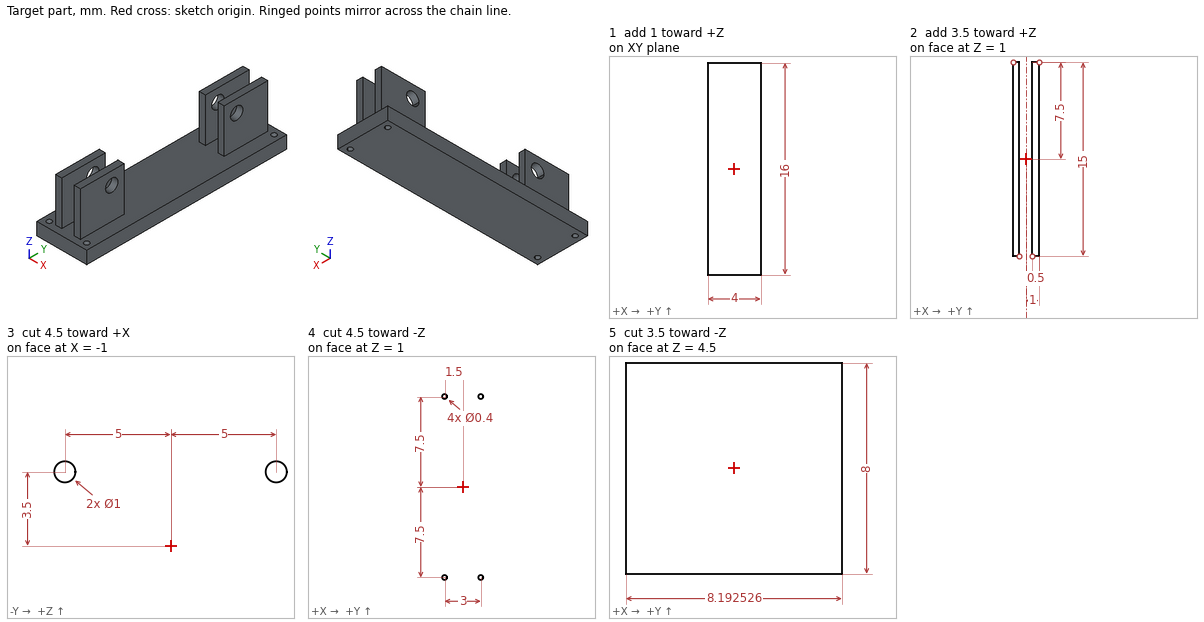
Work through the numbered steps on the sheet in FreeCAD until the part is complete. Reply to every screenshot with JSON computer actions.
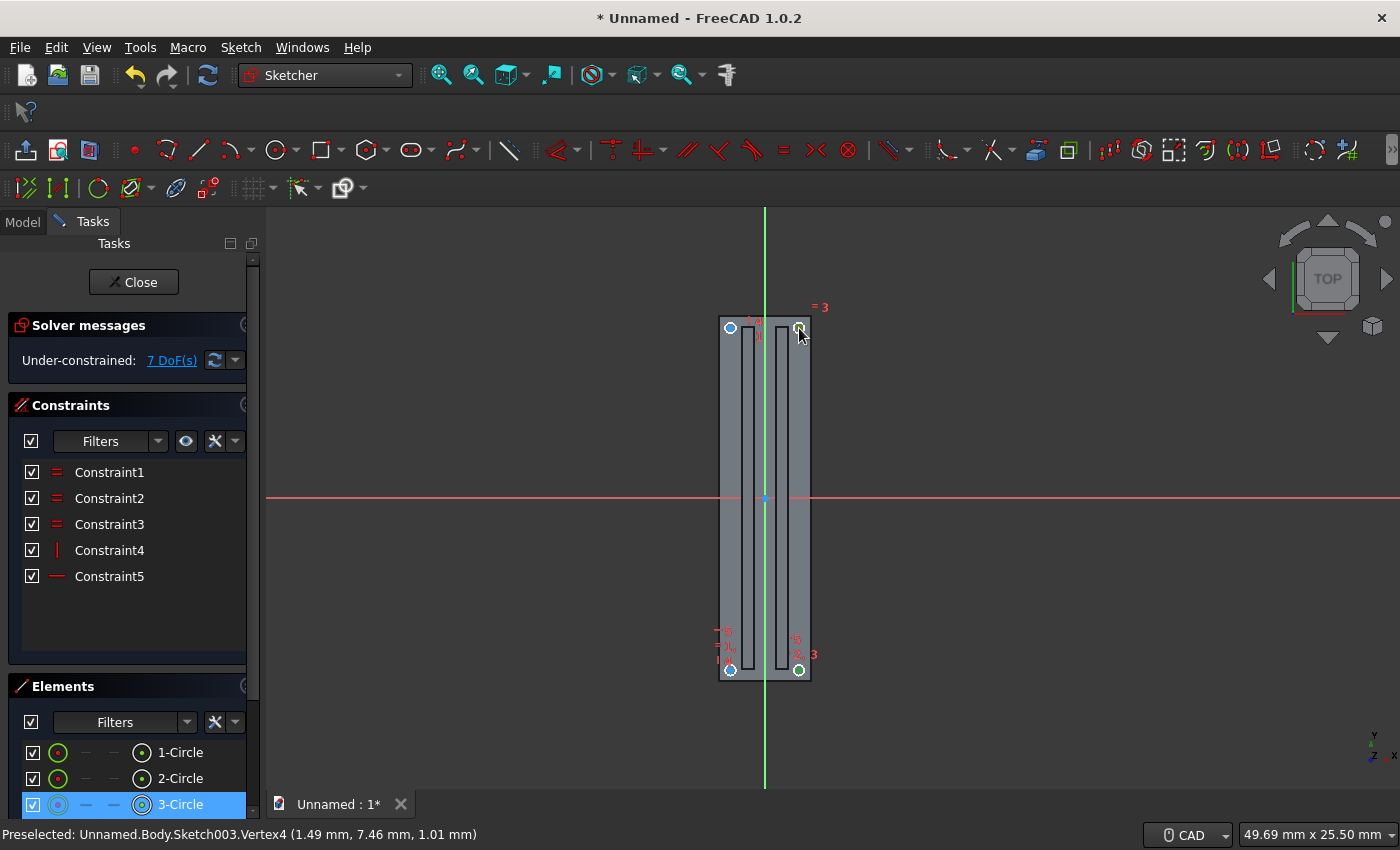
{"action": "key", "text": "v"}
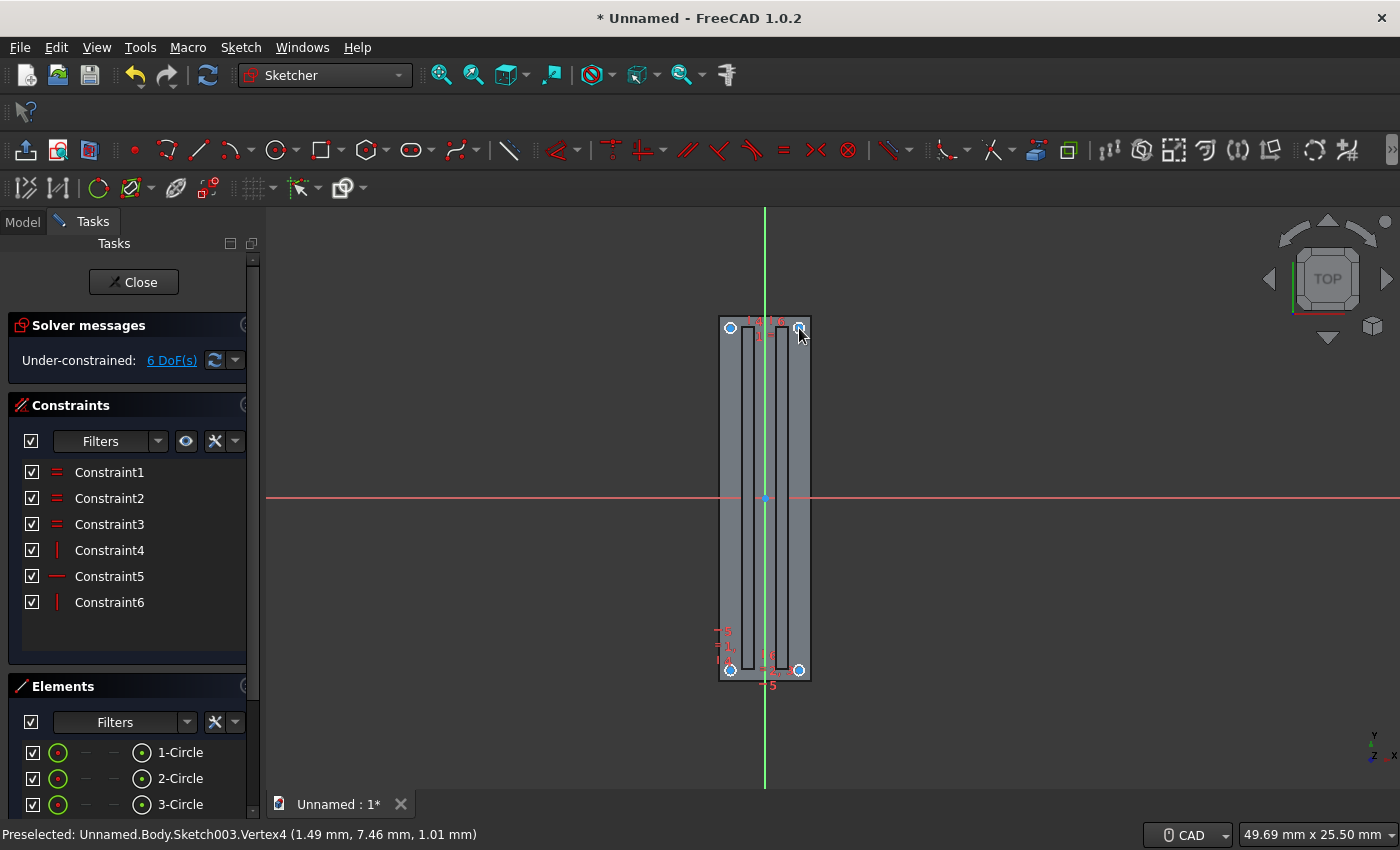
{"action": "left_click", "coordinate": [730, 328]}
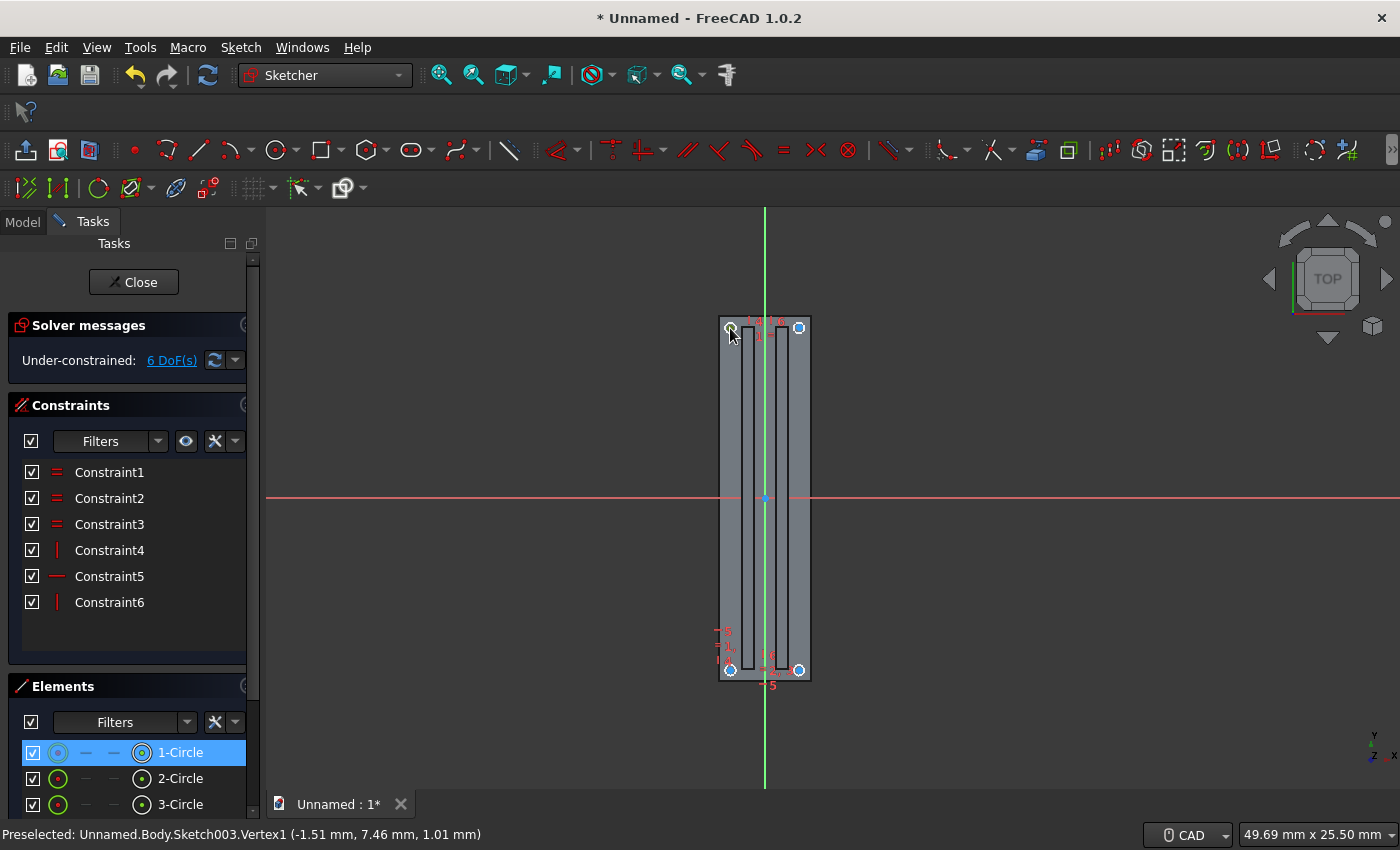
{"action": "left_click", "coordinate": [799, 328]}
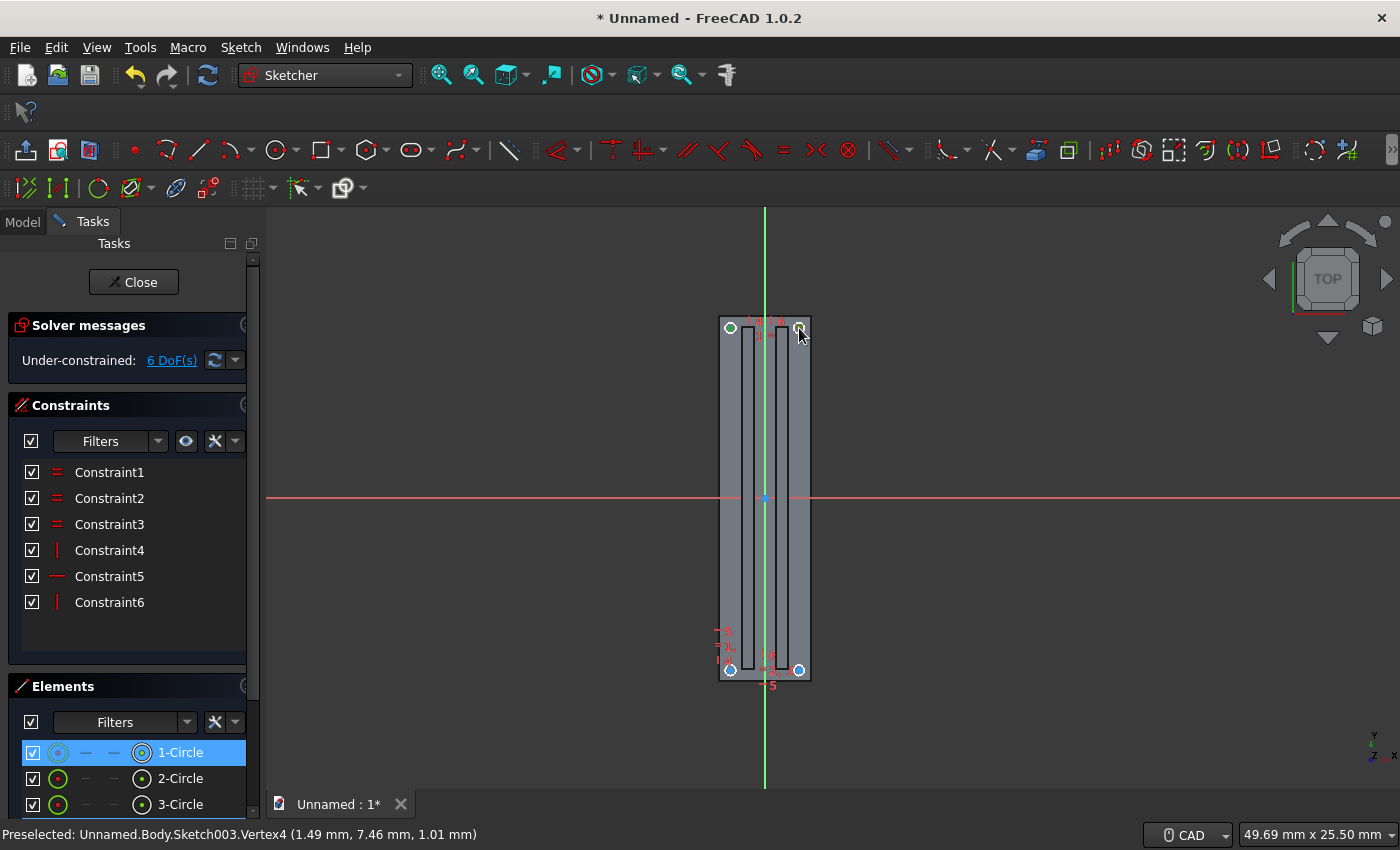
{"action": "left_click", "coordinate": [666, 150]}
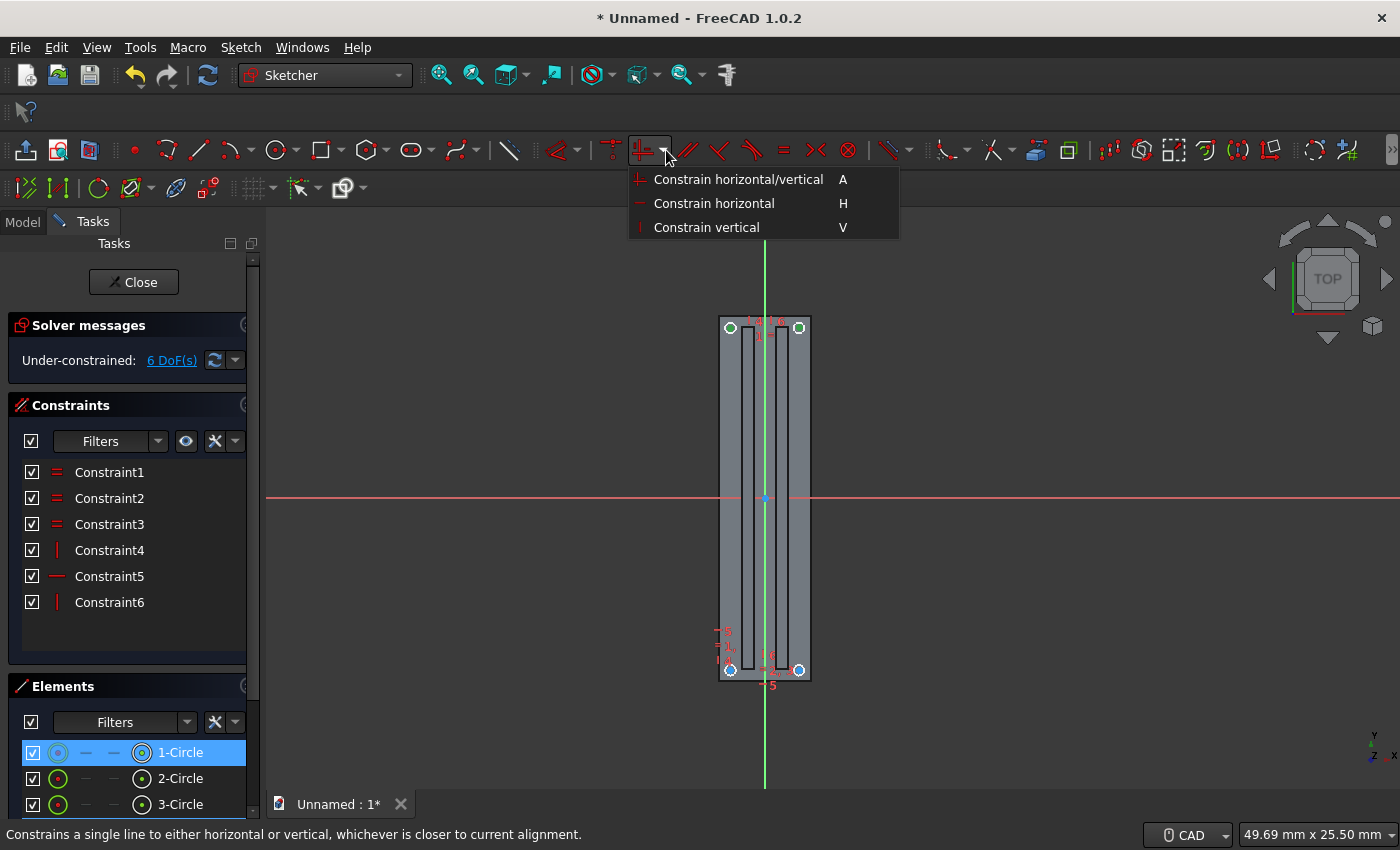
{"action": "left_click", "coordinate": [764, 203]}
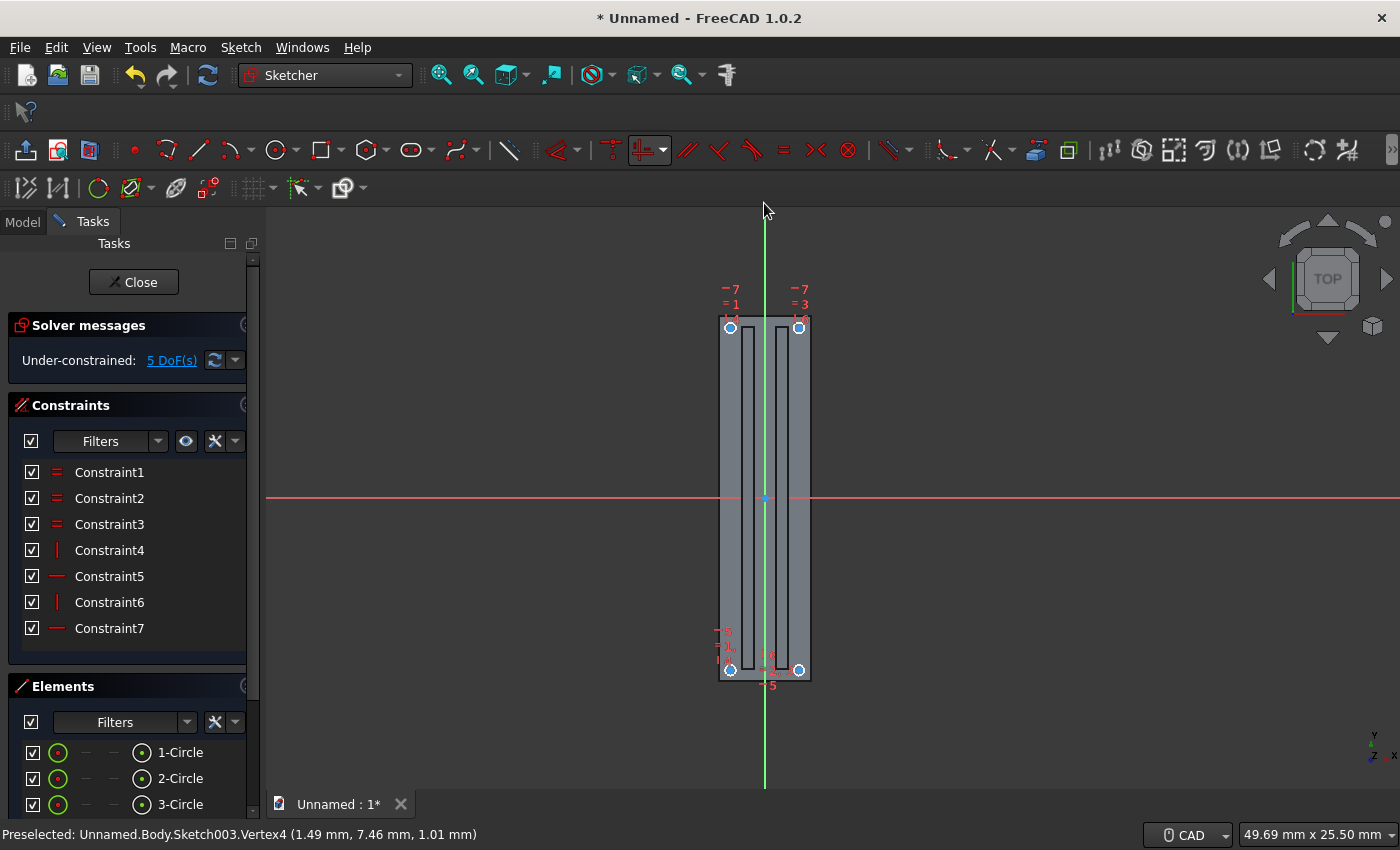
{"action": "key", "text": "d"}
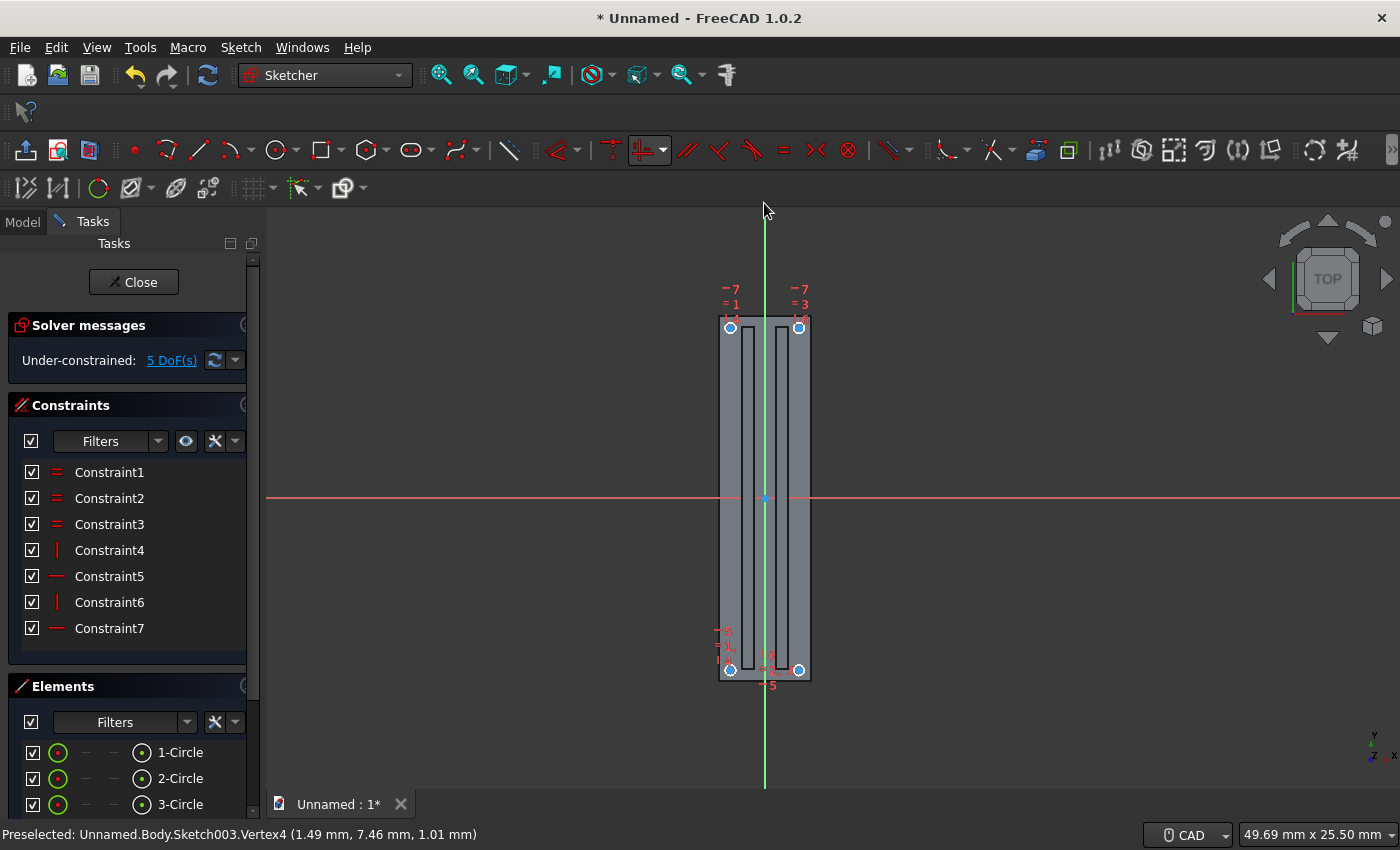
{"action": "scroll", "coordinate": [734, 324], "scroll_direction": "up", "scroll_amount": 8}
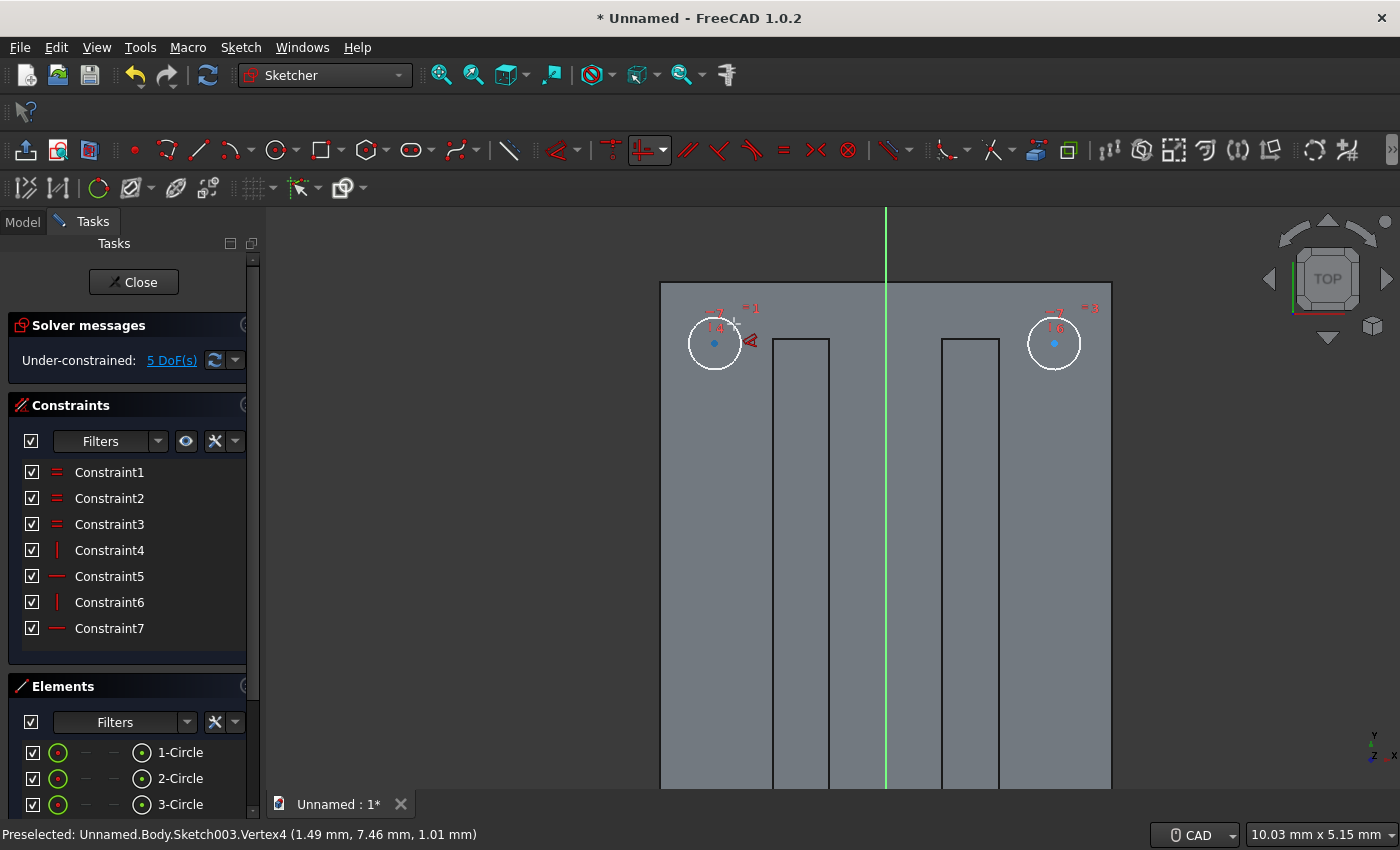
{"action": "left_click", "coordinate": [733, 325]}
{"action": "left_click", "coordinate": [755, 302]}